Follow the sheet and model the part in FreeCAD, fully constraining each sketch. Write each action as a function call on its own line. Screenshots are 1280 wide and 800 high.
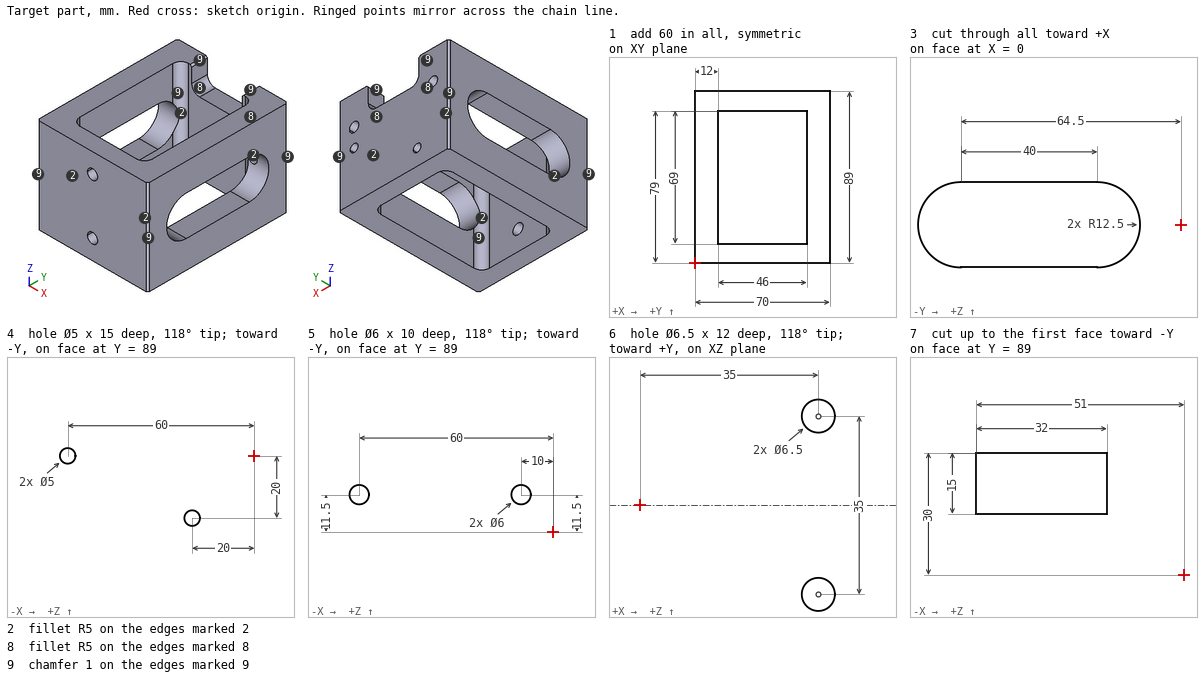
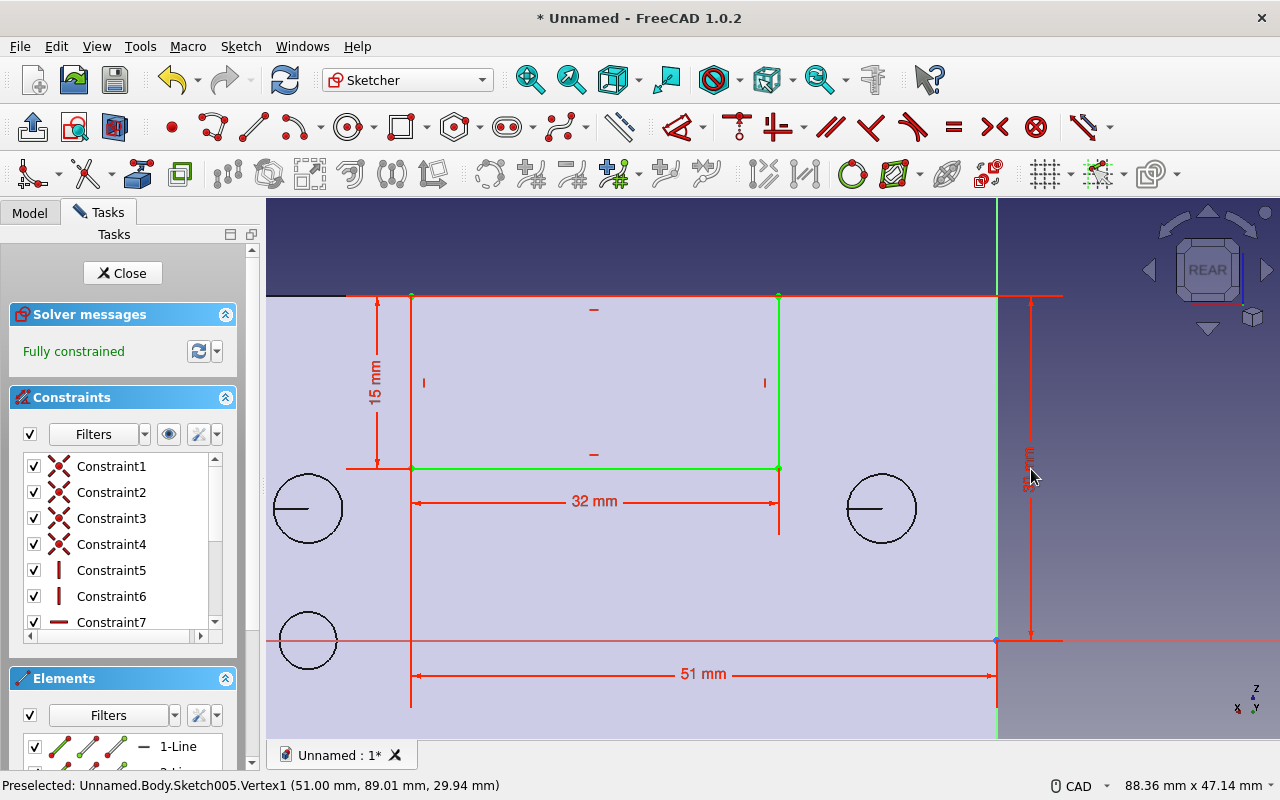
click(123, 273)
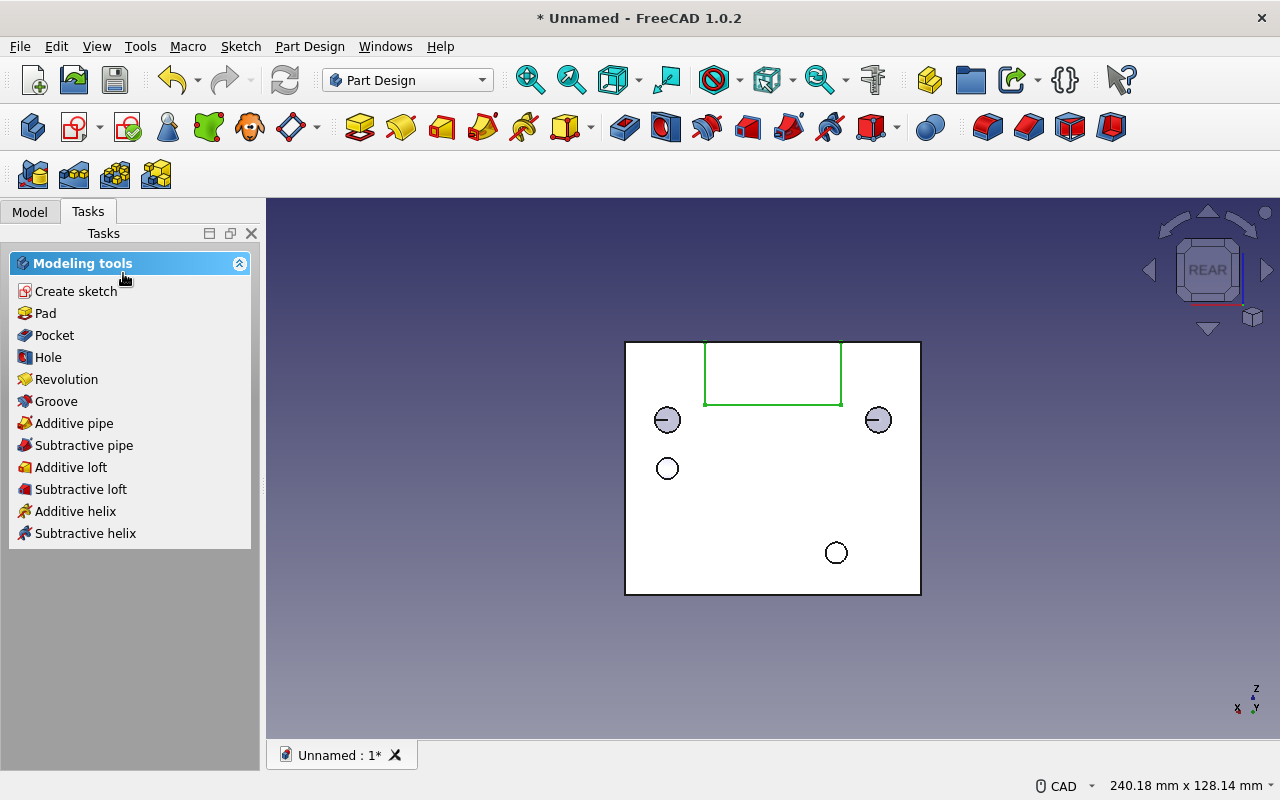
click(625, 128)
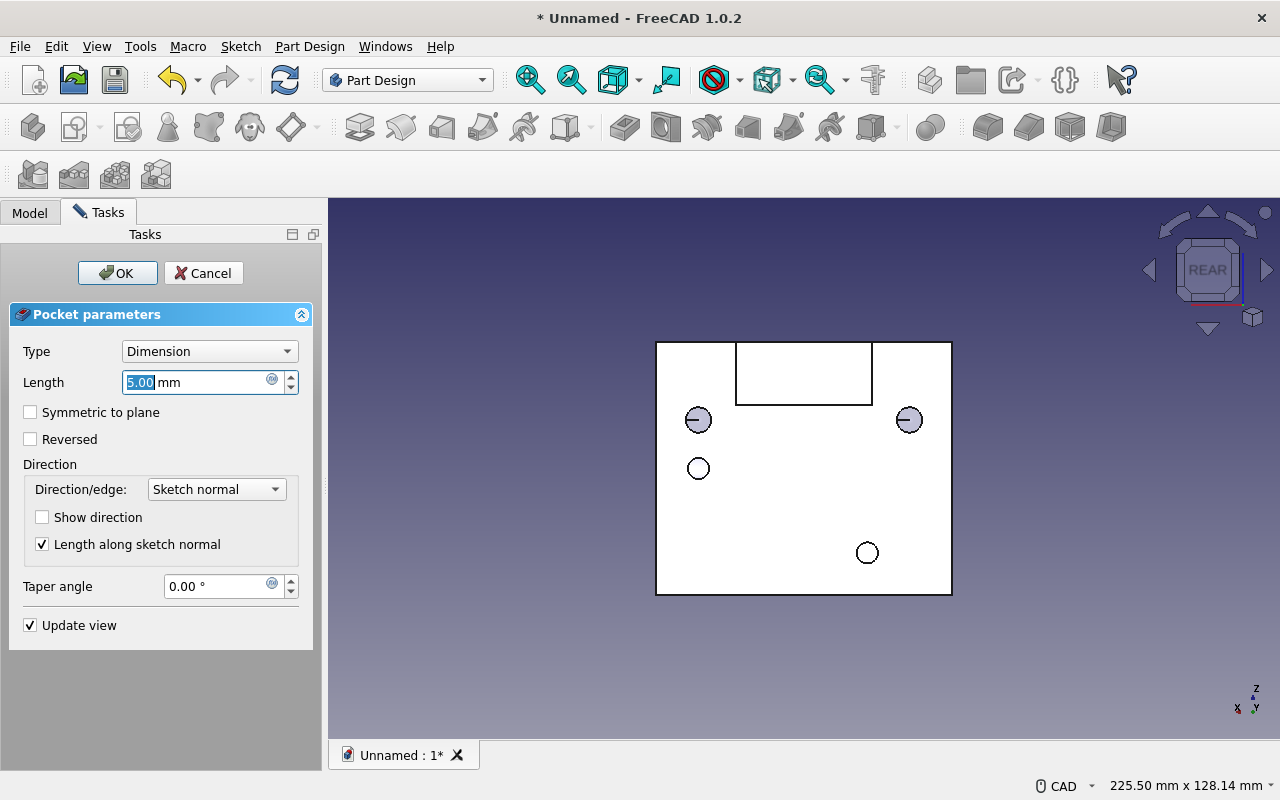
click(210, 352)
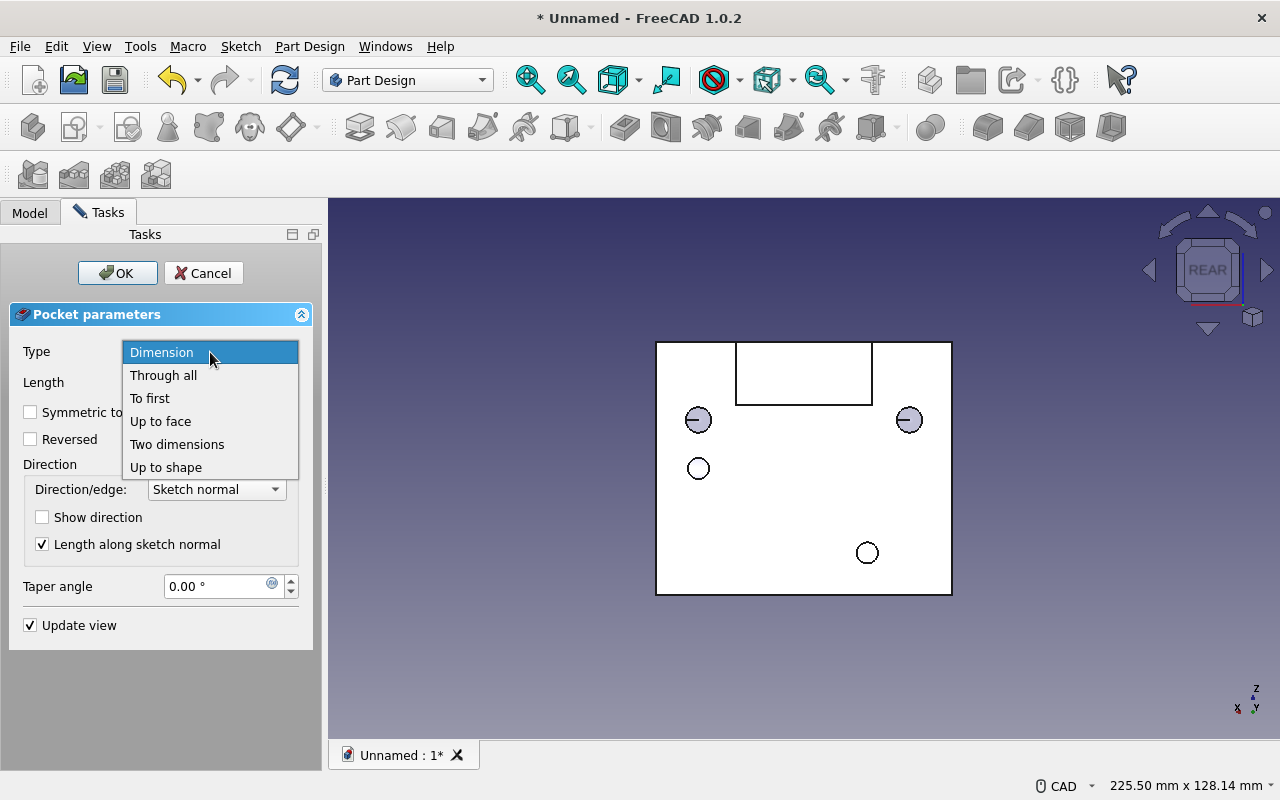
click(208, 398)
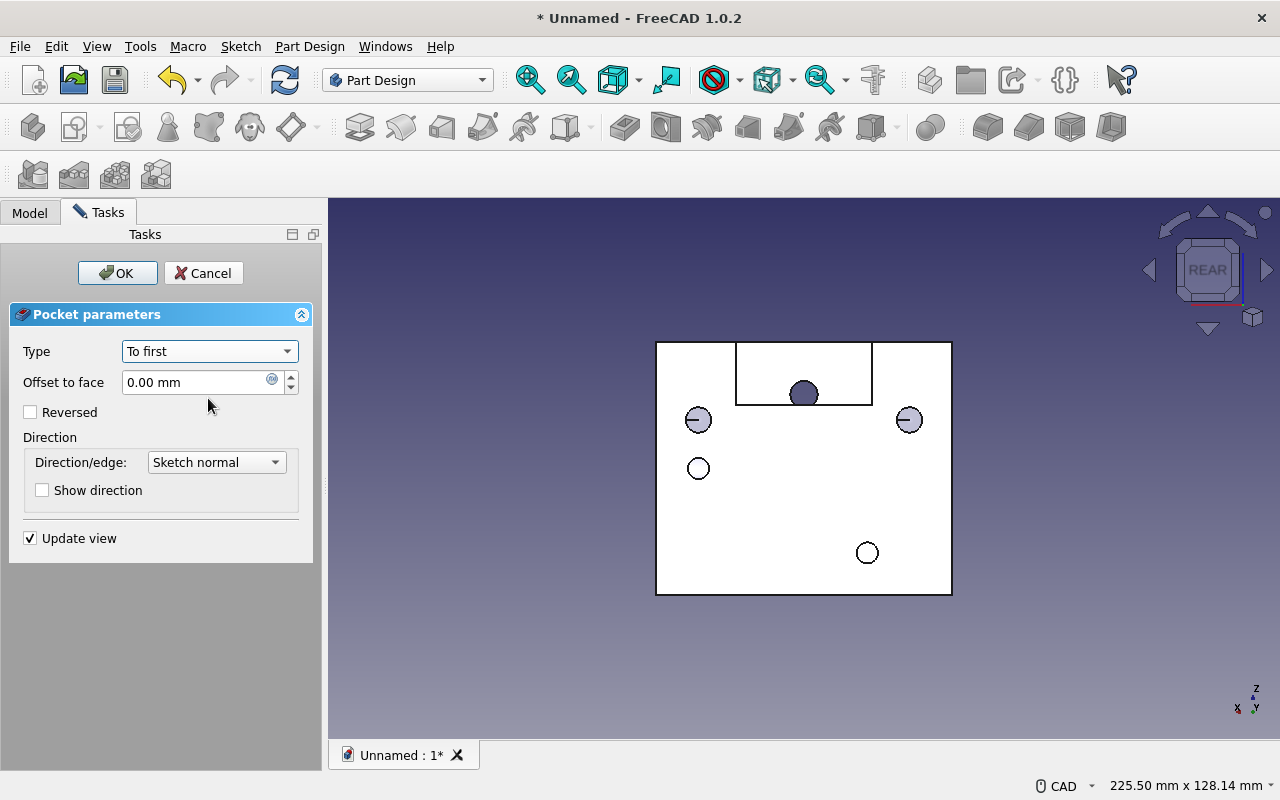
click(118, 273)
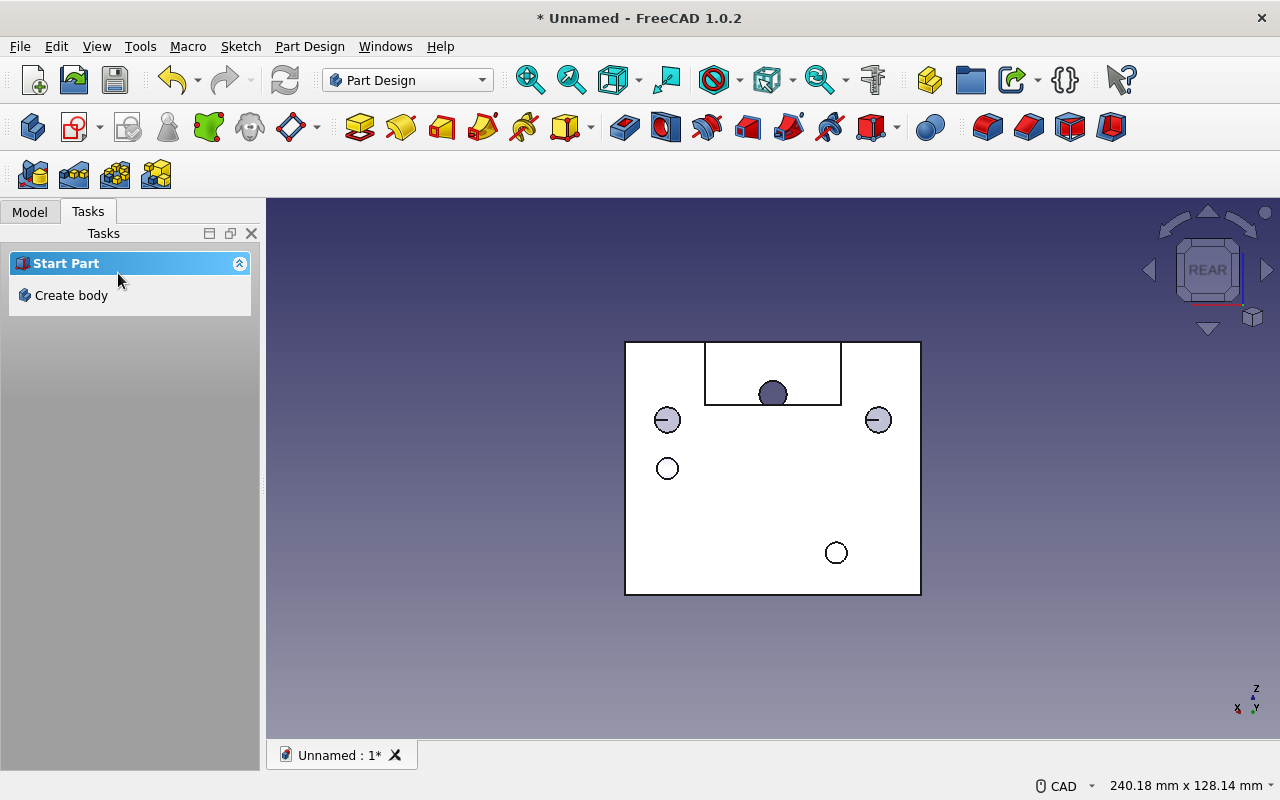
key(0)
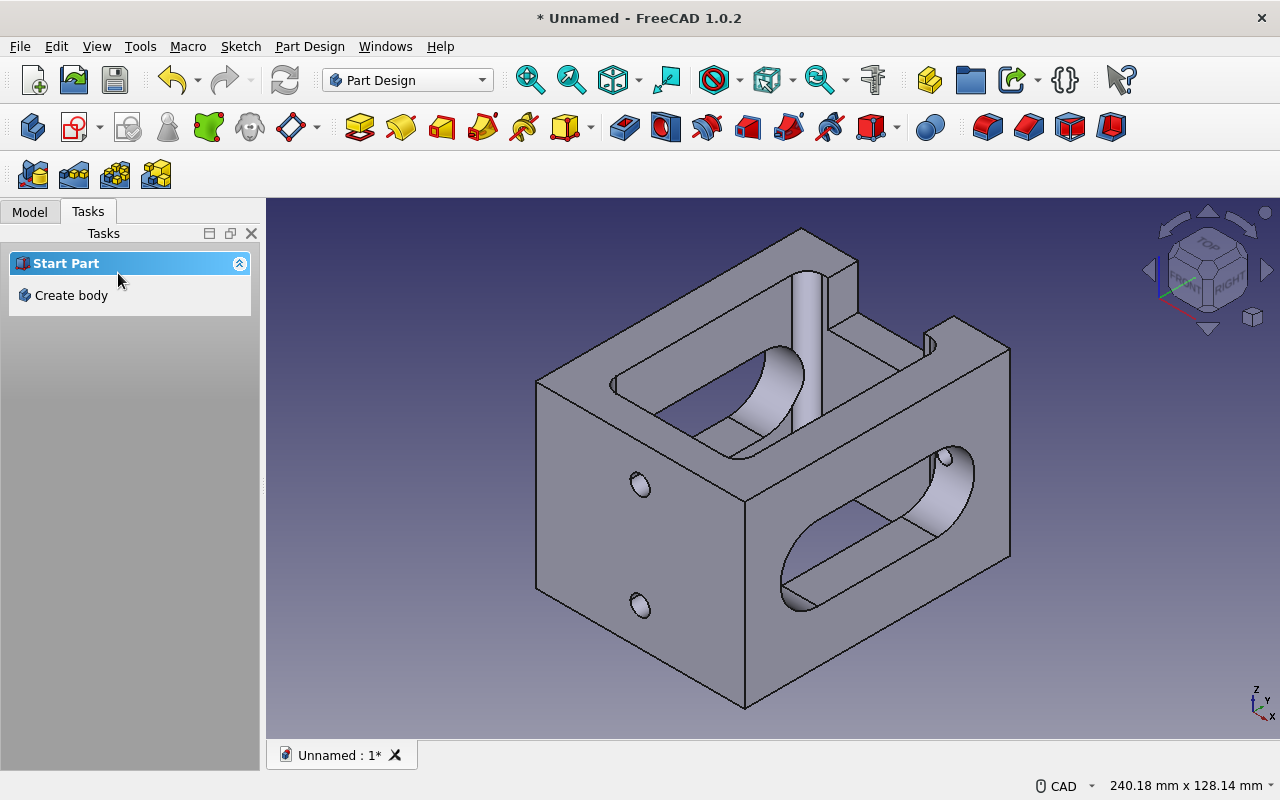
key(2)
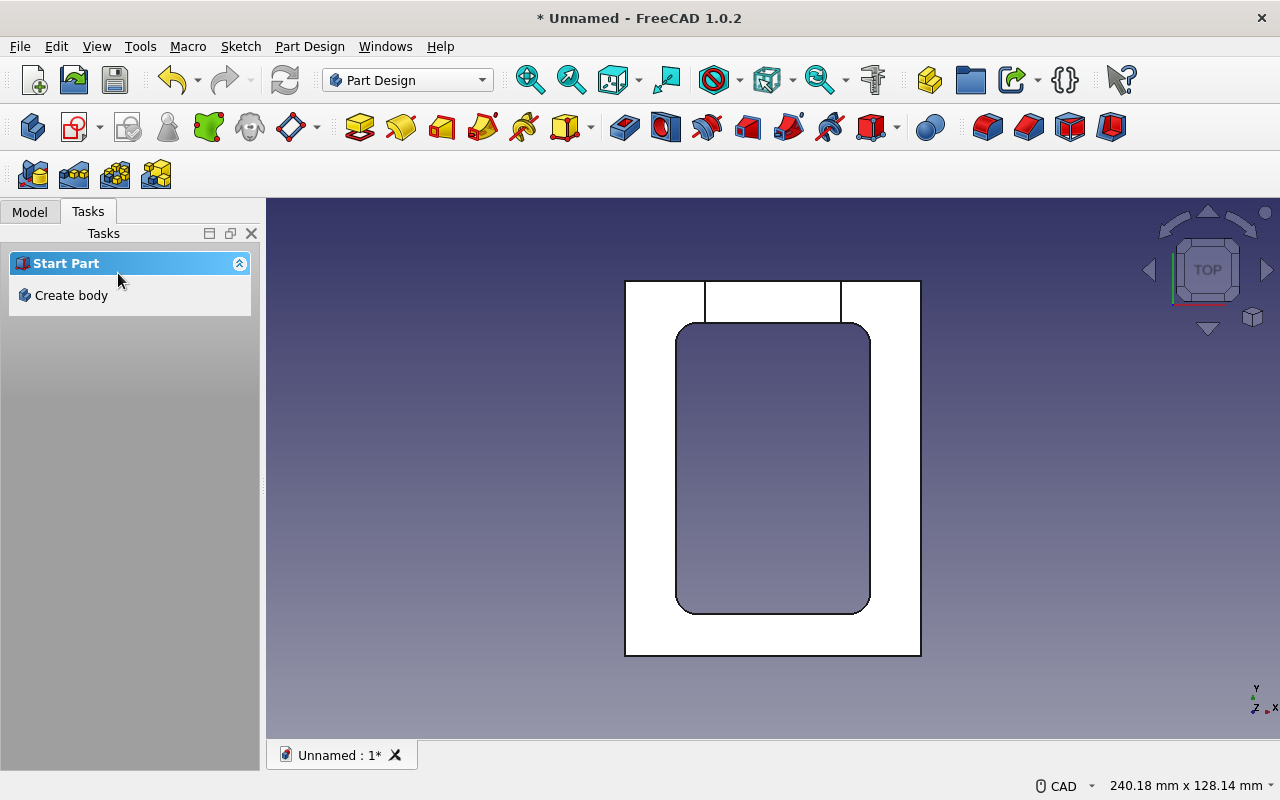
key(1)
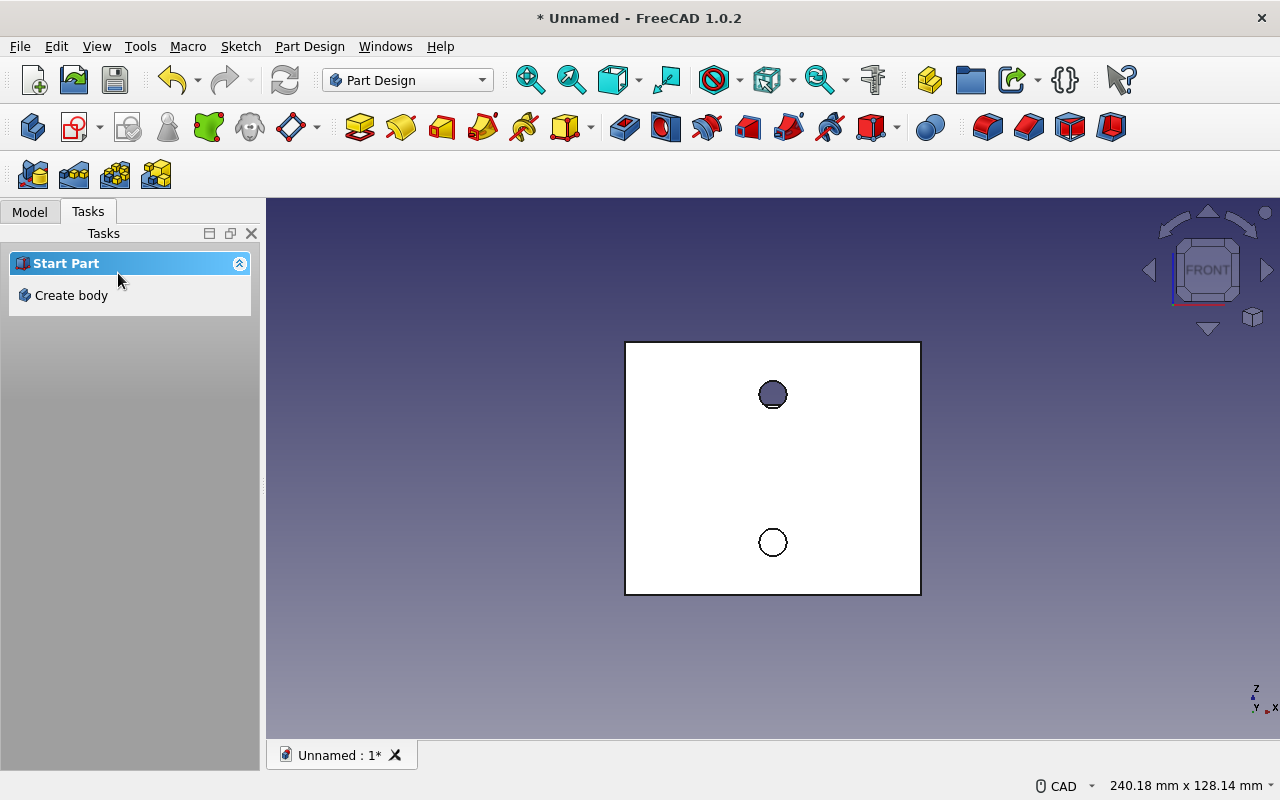
key(3)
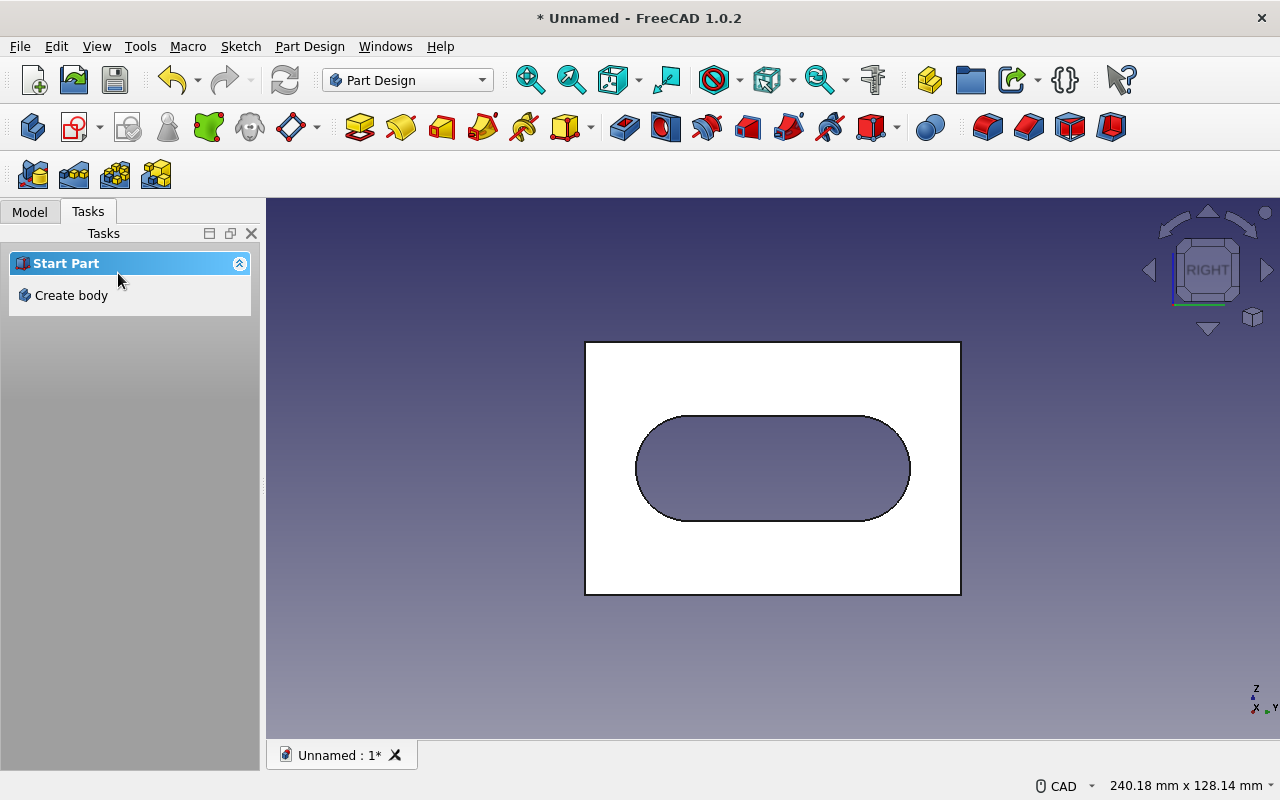
key(5)